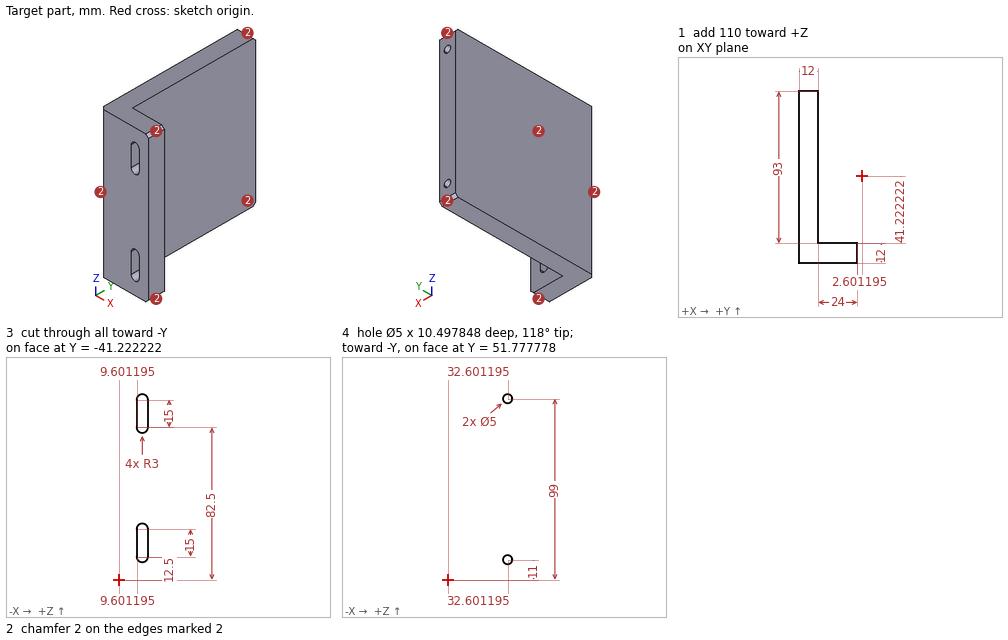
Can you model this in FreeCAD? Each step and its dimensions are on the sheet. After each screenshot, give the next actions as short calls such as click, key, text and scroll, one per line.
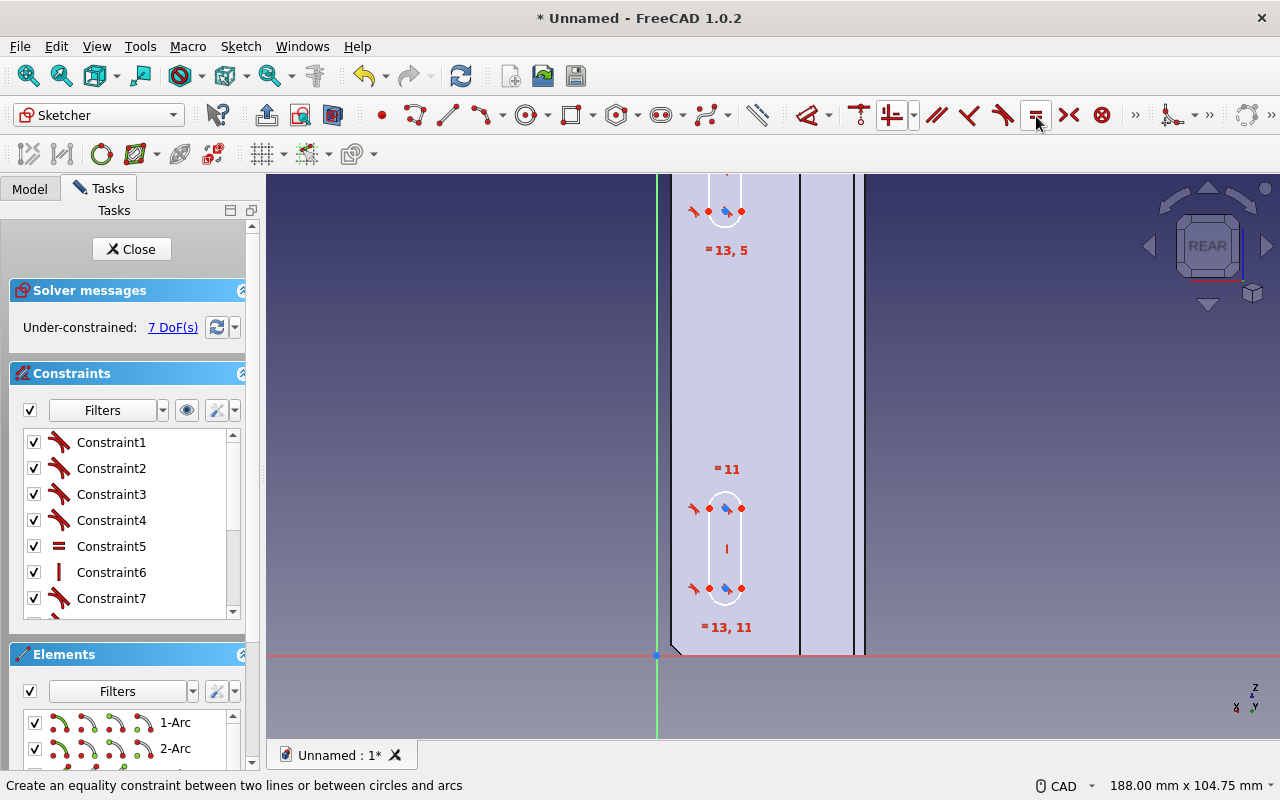
click(806, 116)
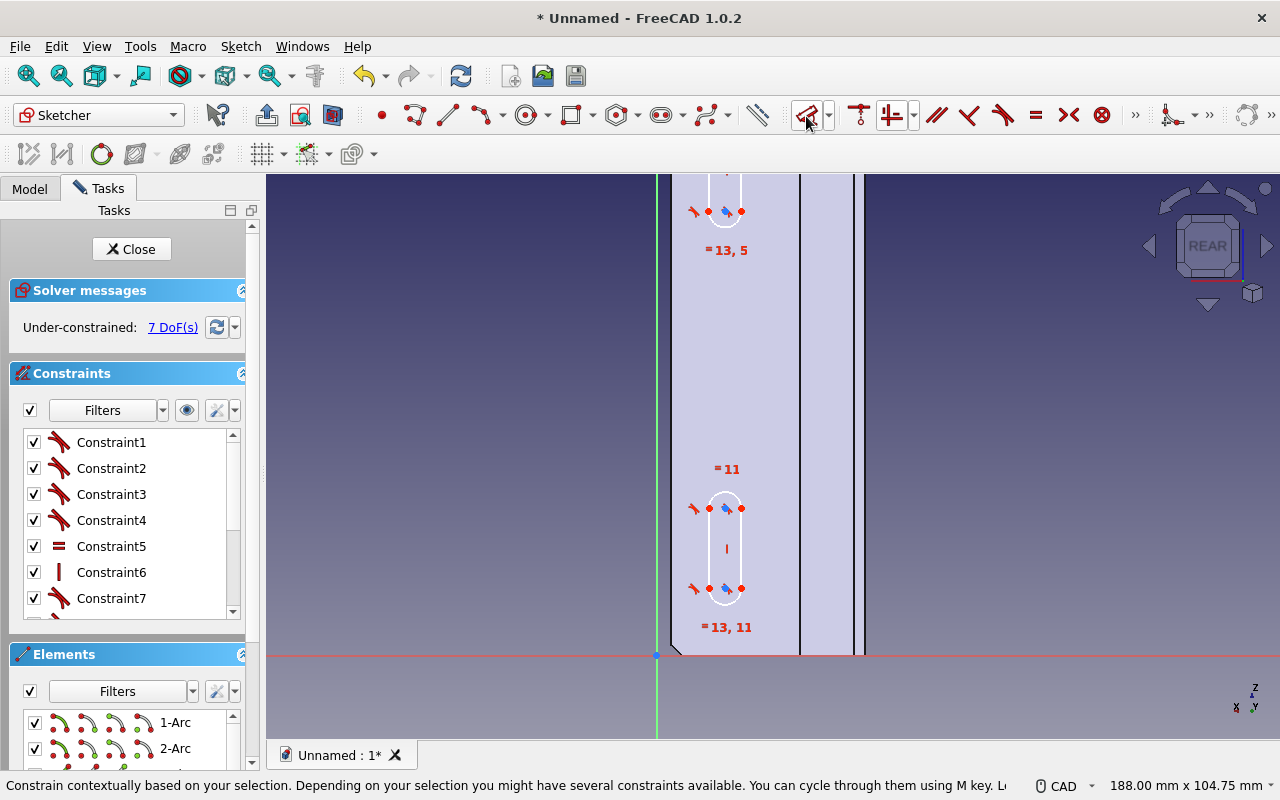
scroll(716, 224, up, 5)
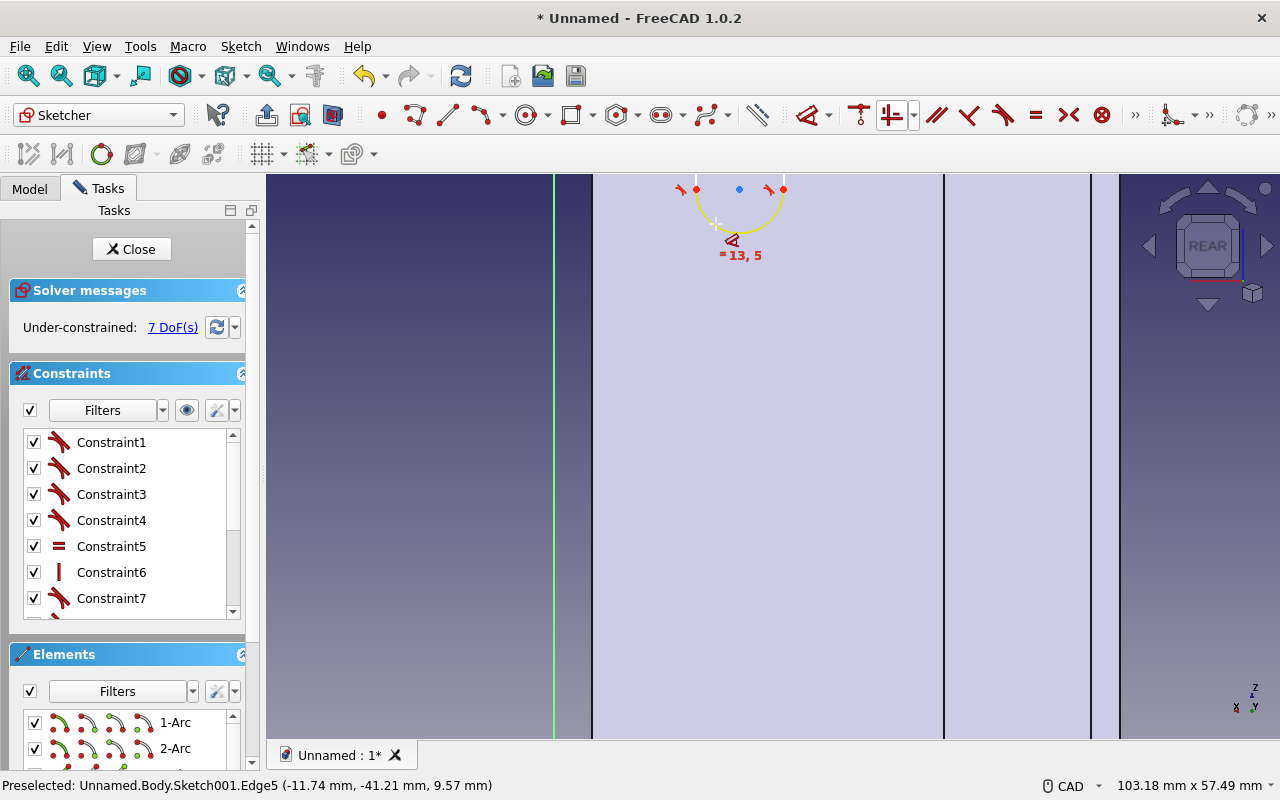
click(714, 225)
click(695, 251)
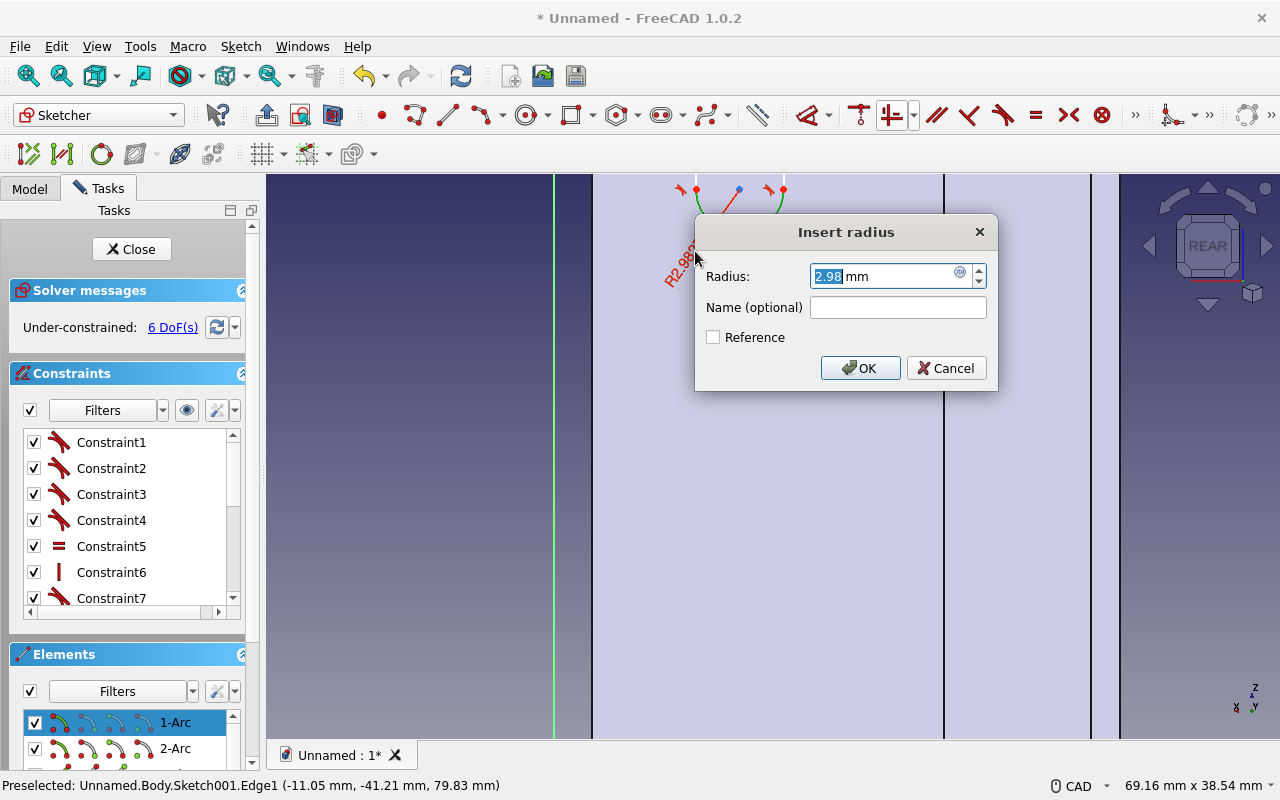
text(3)
key(Return)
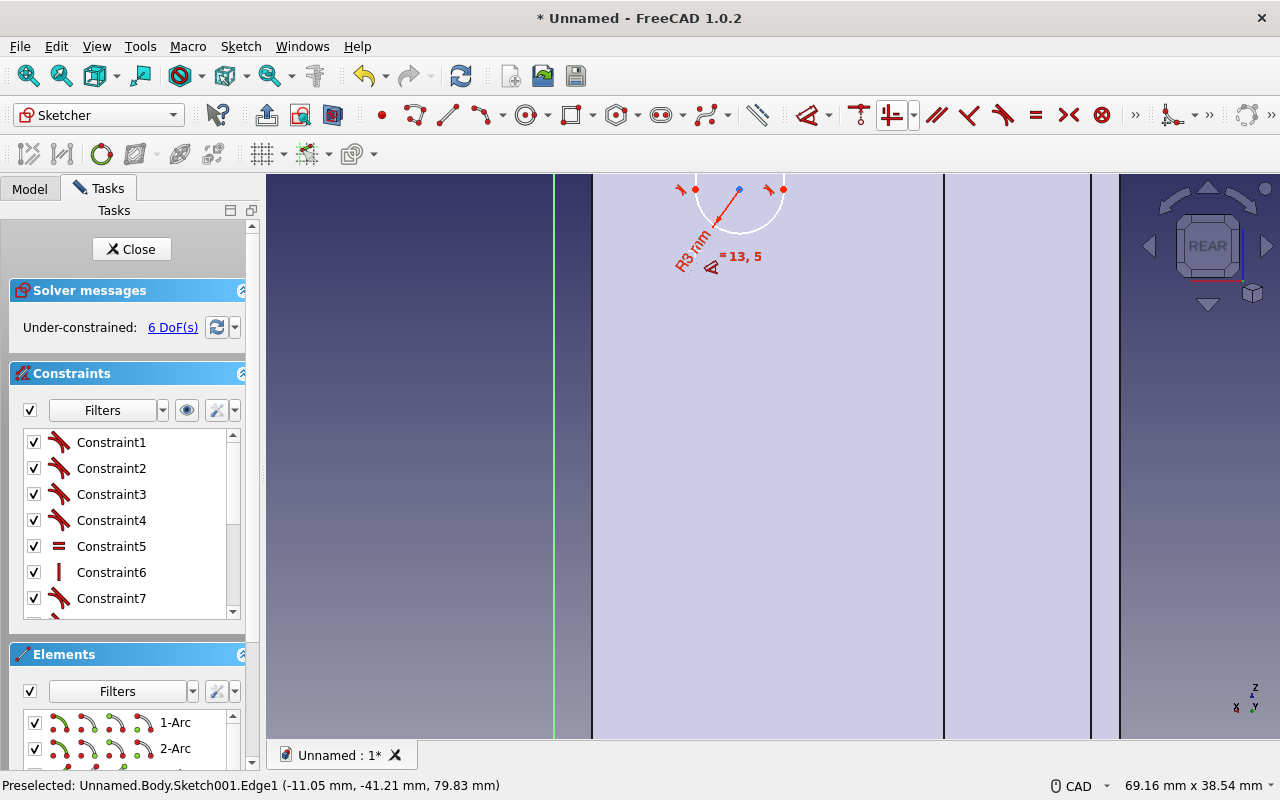
scroll(716, 390, down, 7)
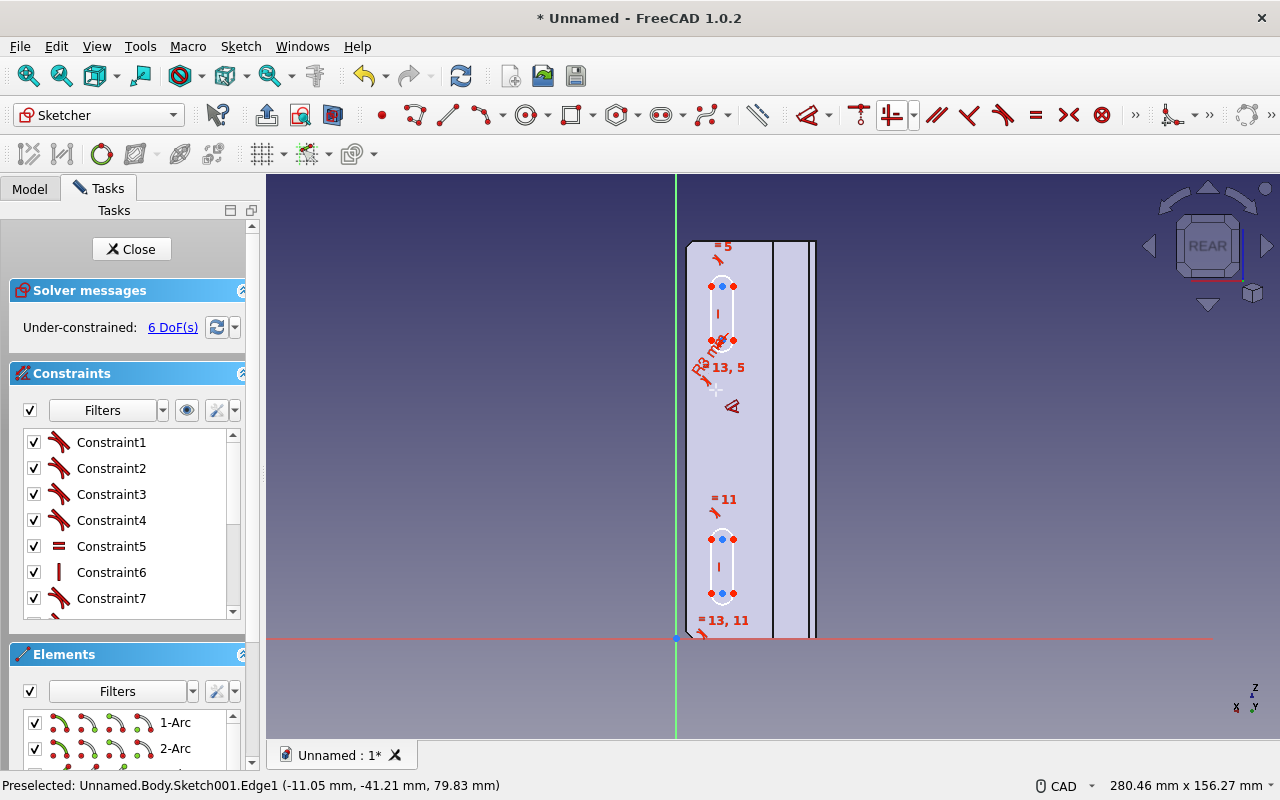
click(711, 325)
click(769, 314)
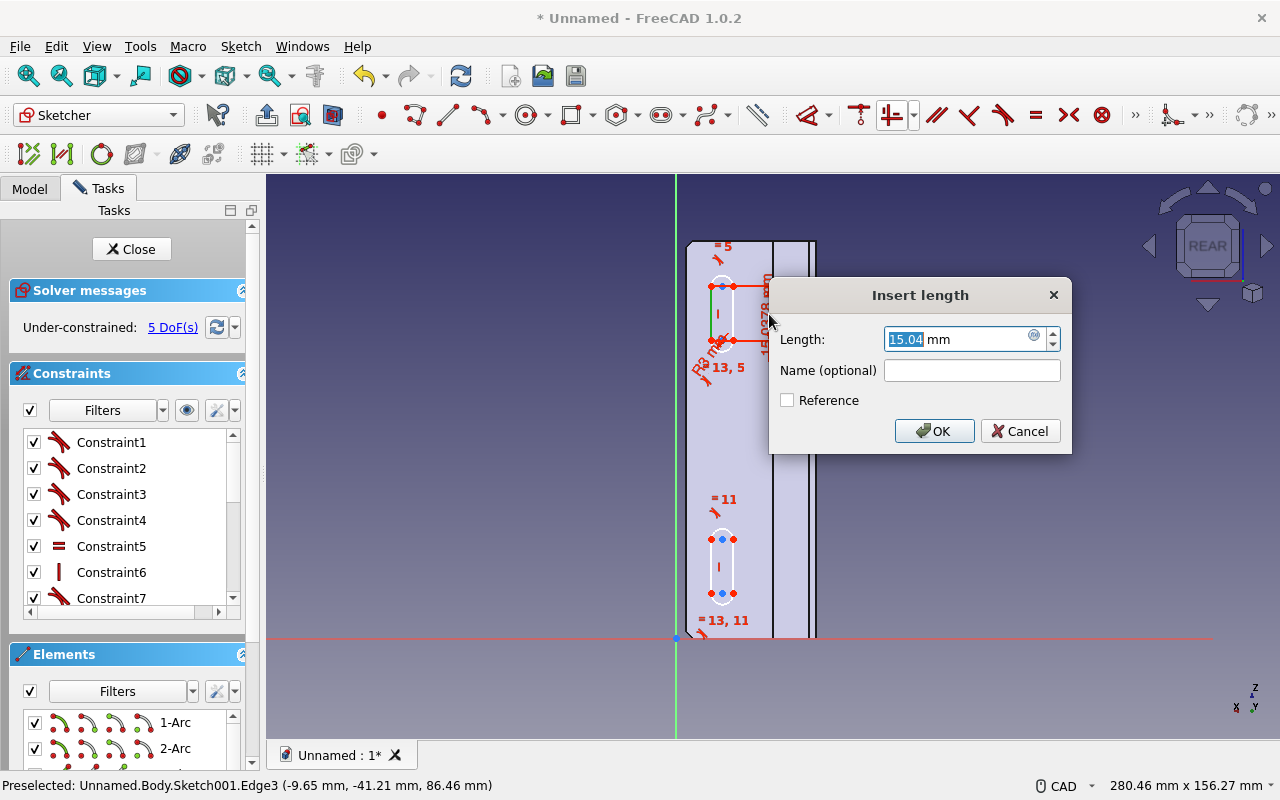
text(15)
key(Return)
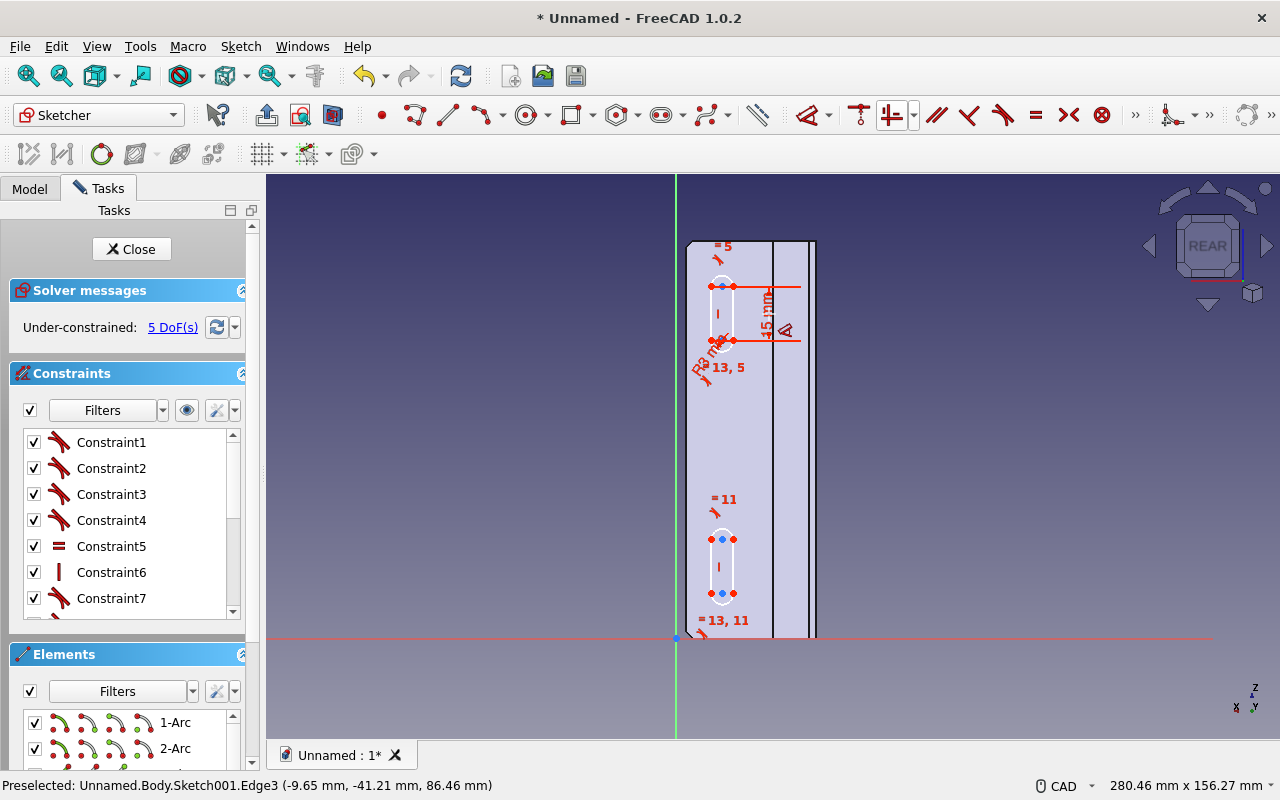
click(711, 578)
click(769, 567)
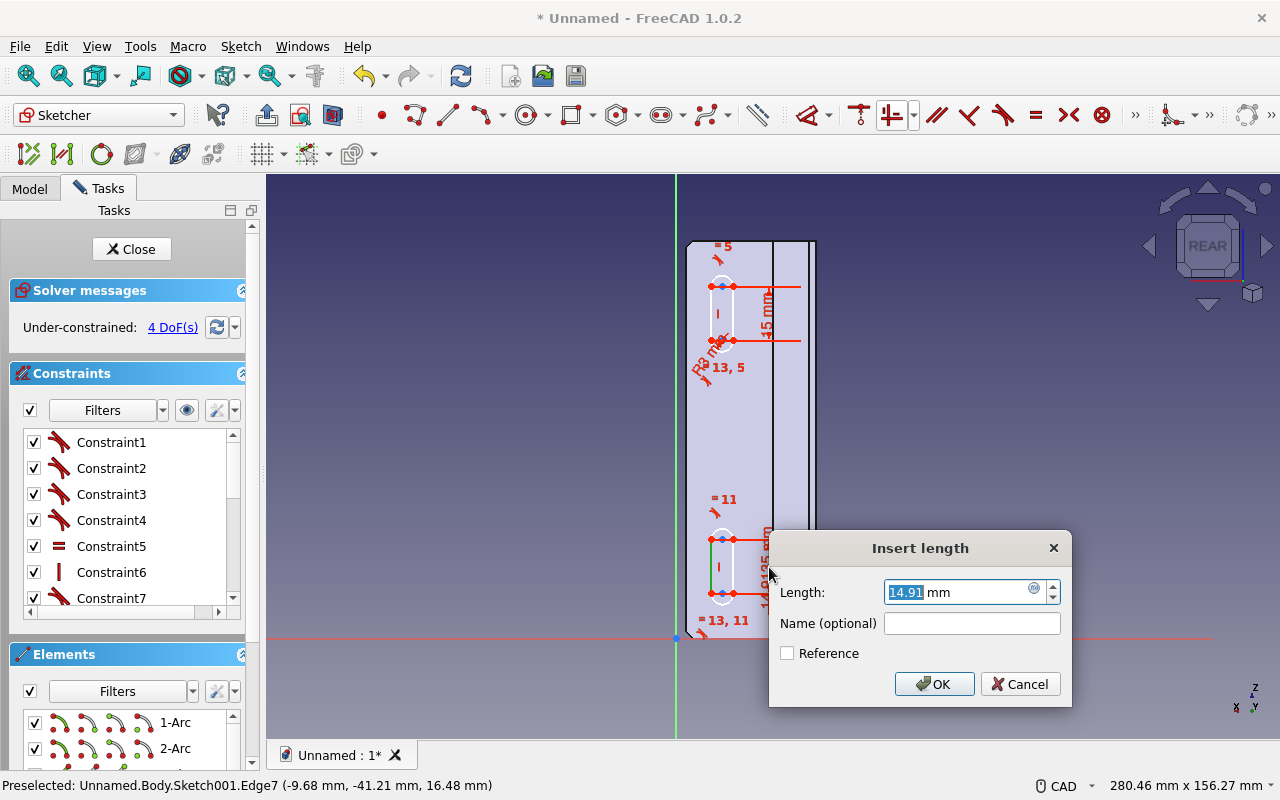
text(15)
key(Return)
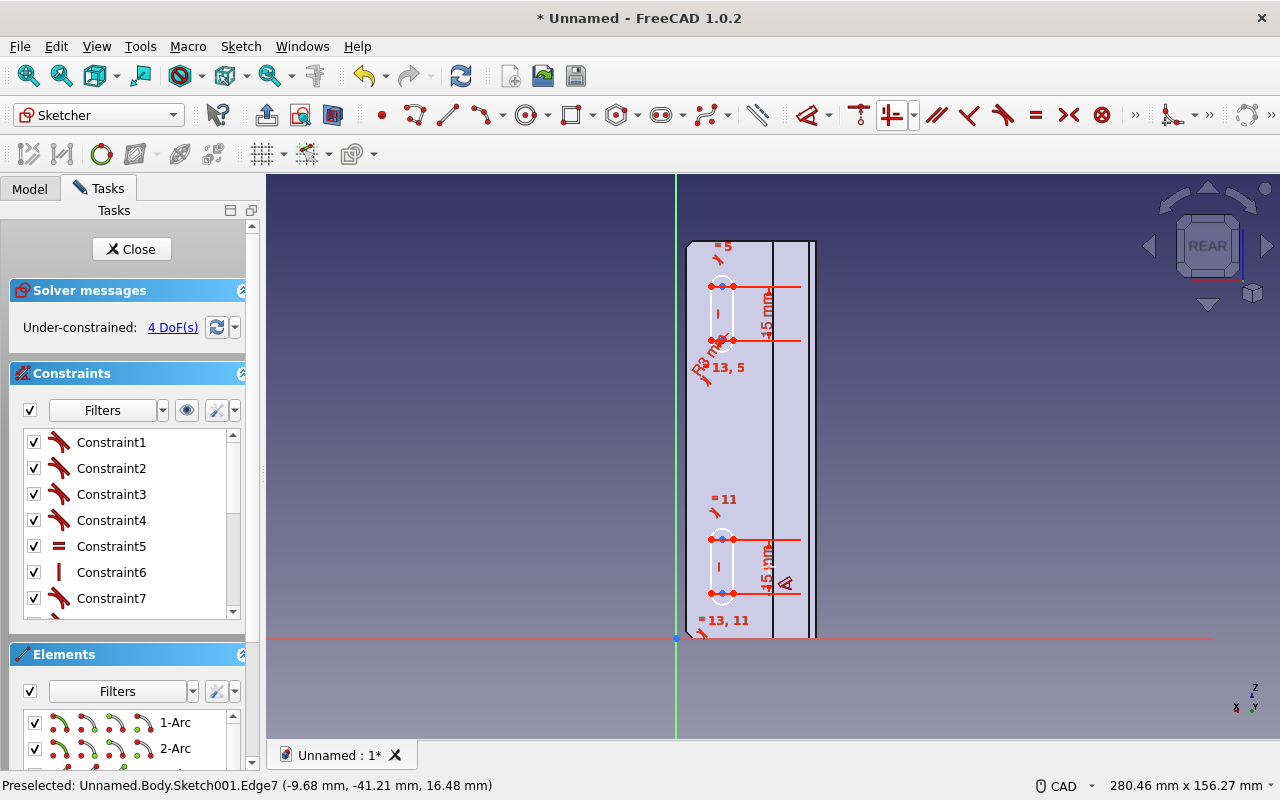
click(711, 341)
click(642, 490)